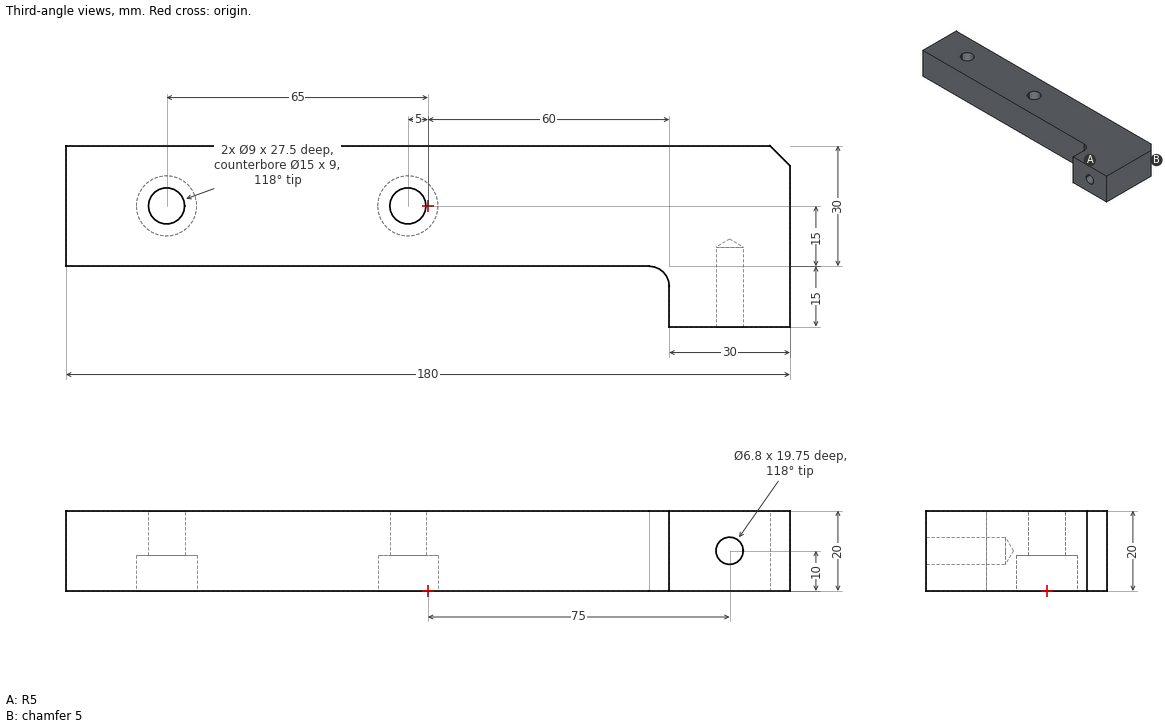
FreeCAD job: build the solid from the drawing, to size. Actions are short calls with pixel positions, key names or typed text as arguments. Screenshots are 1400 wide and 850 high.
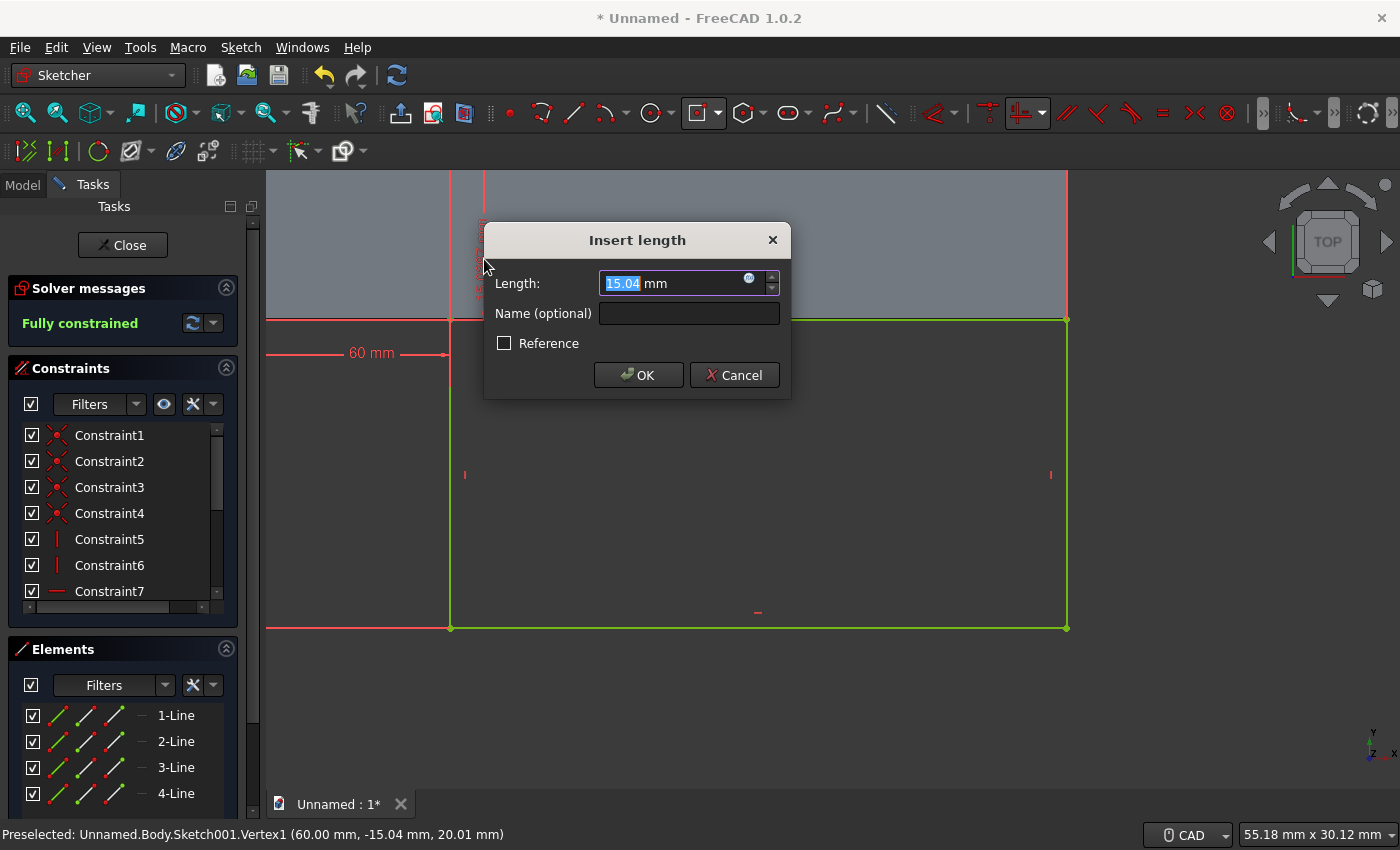
text(15)
key(Return)
key(Escape)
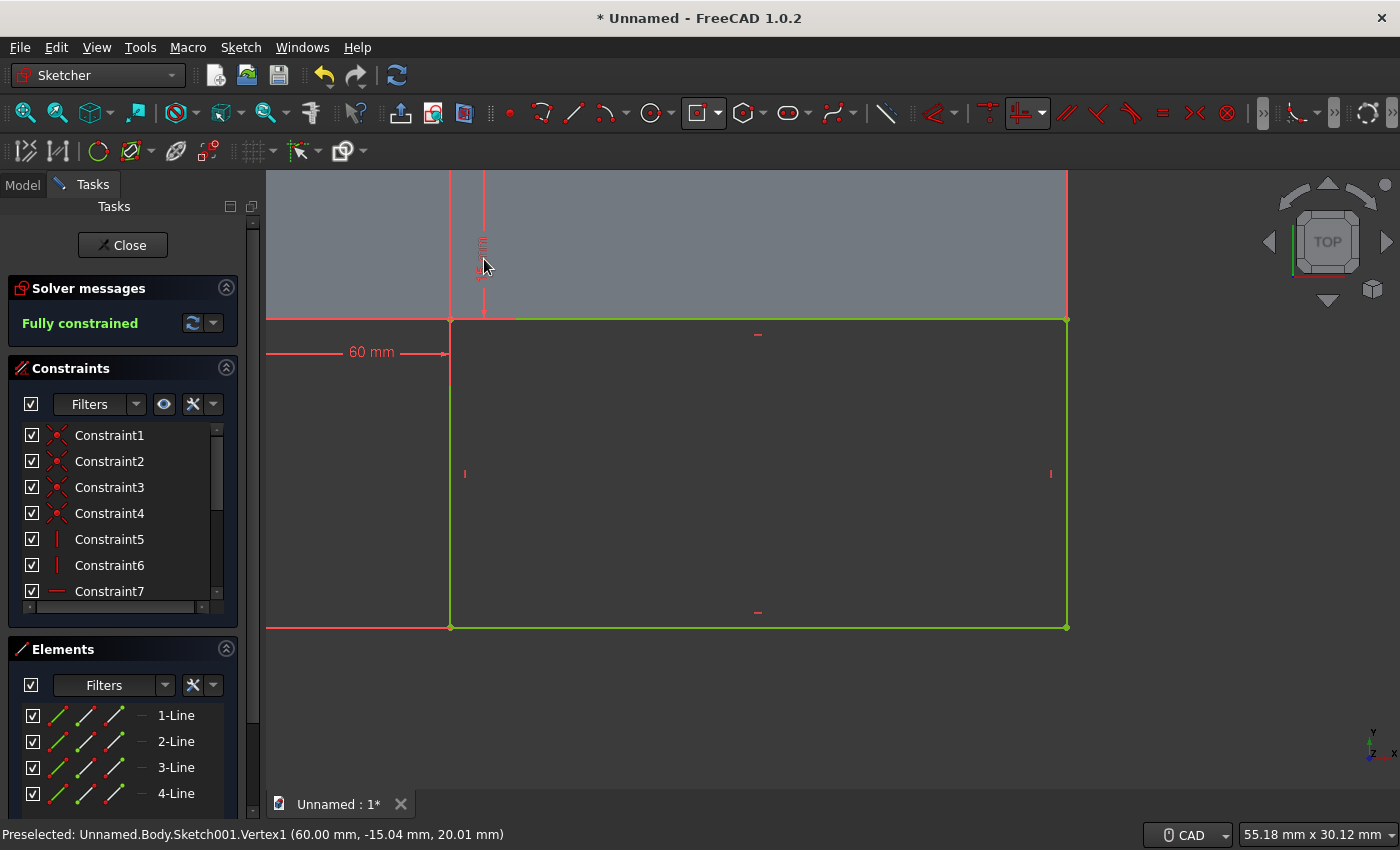
click(123, 245)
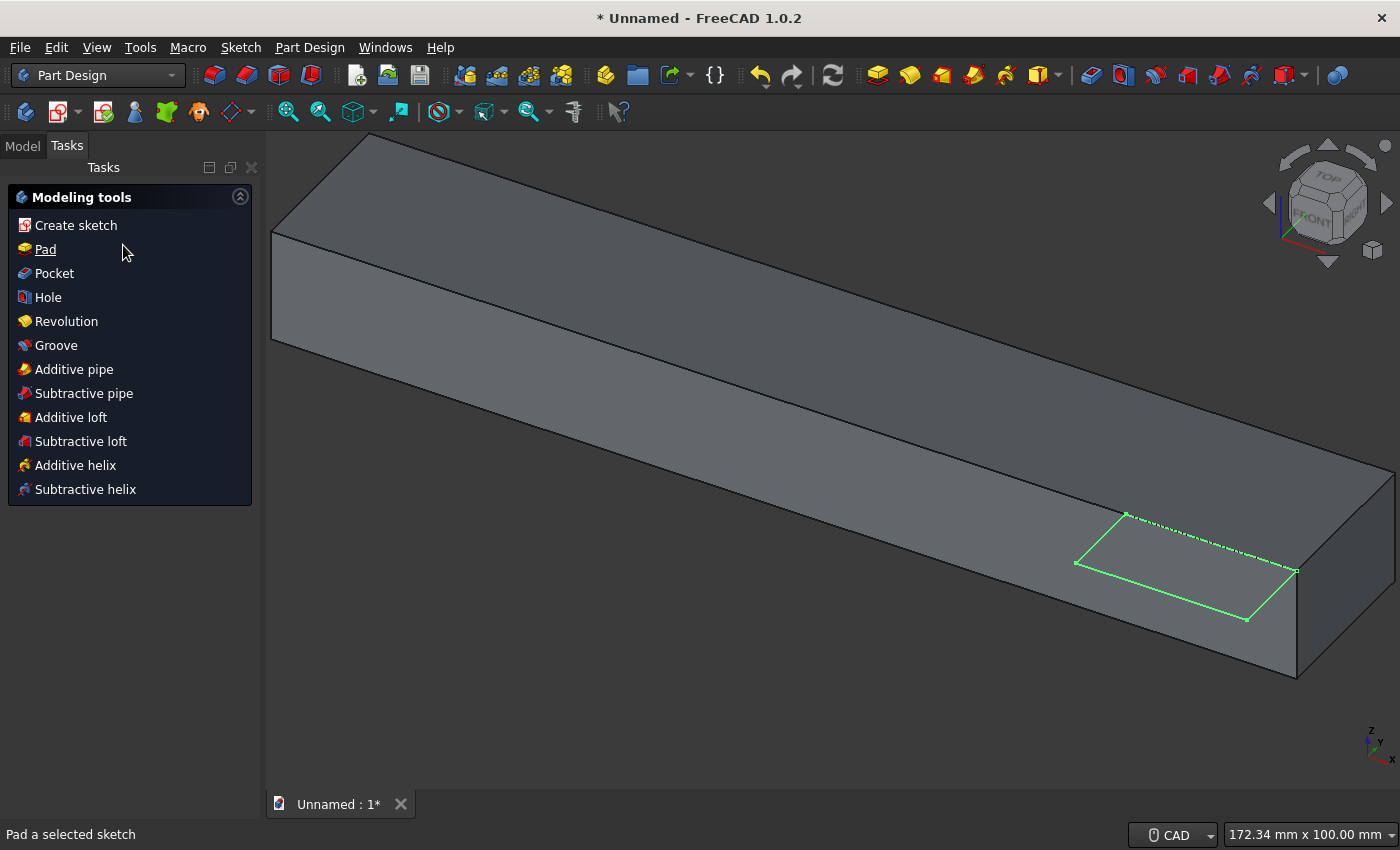
click(878, 76)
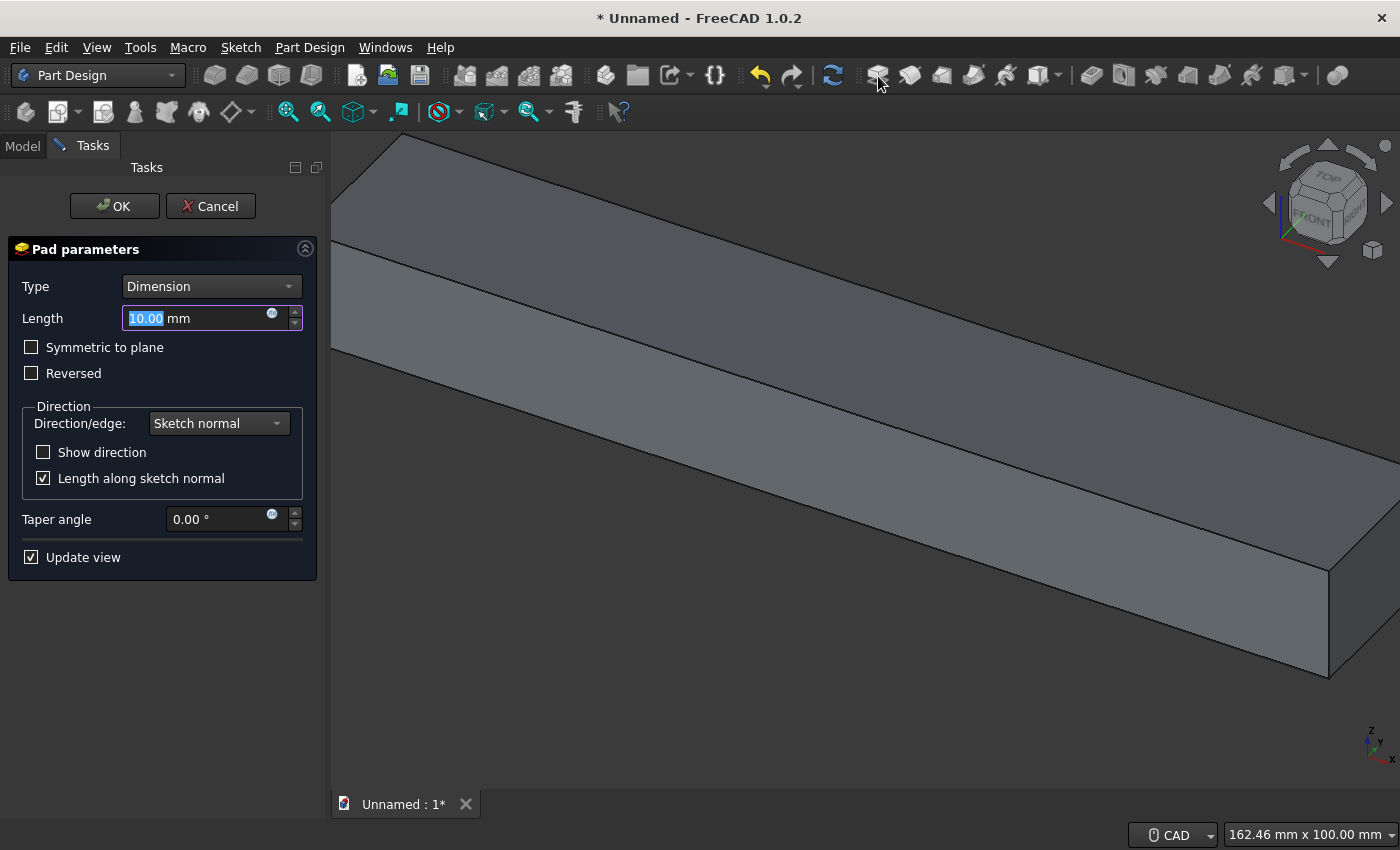
text(20)
key(Tab)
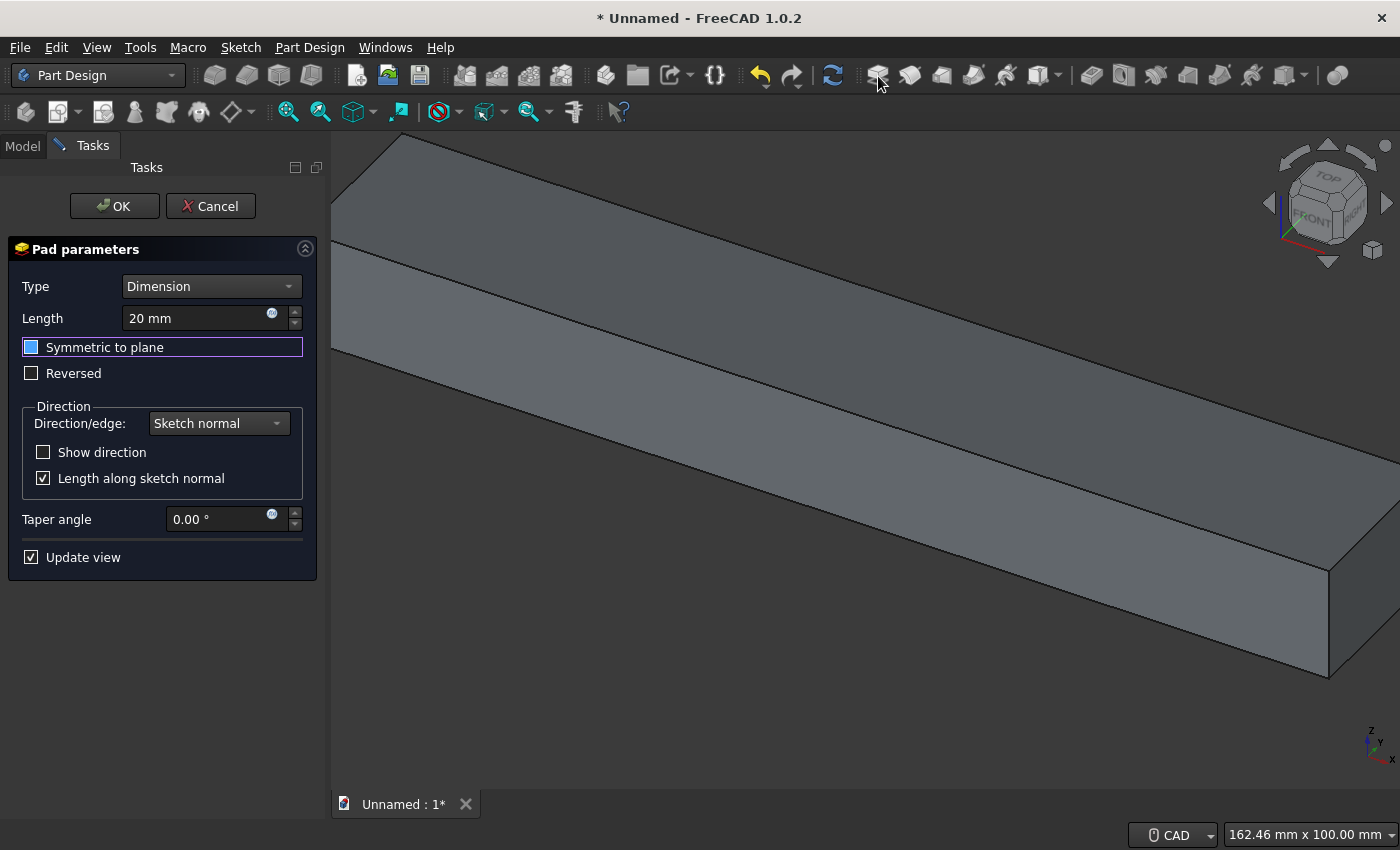
click(30, 373)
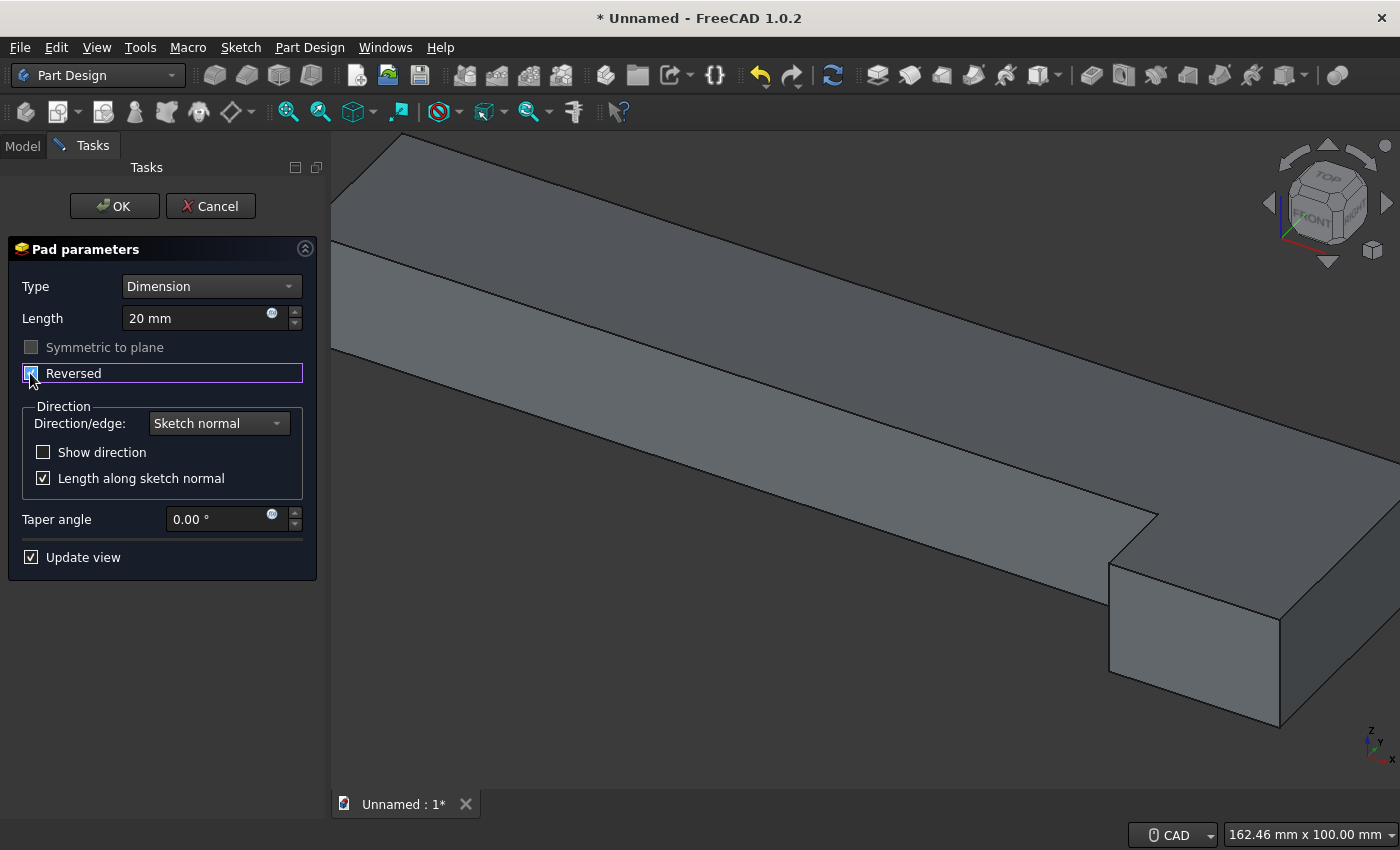
click(115, 206)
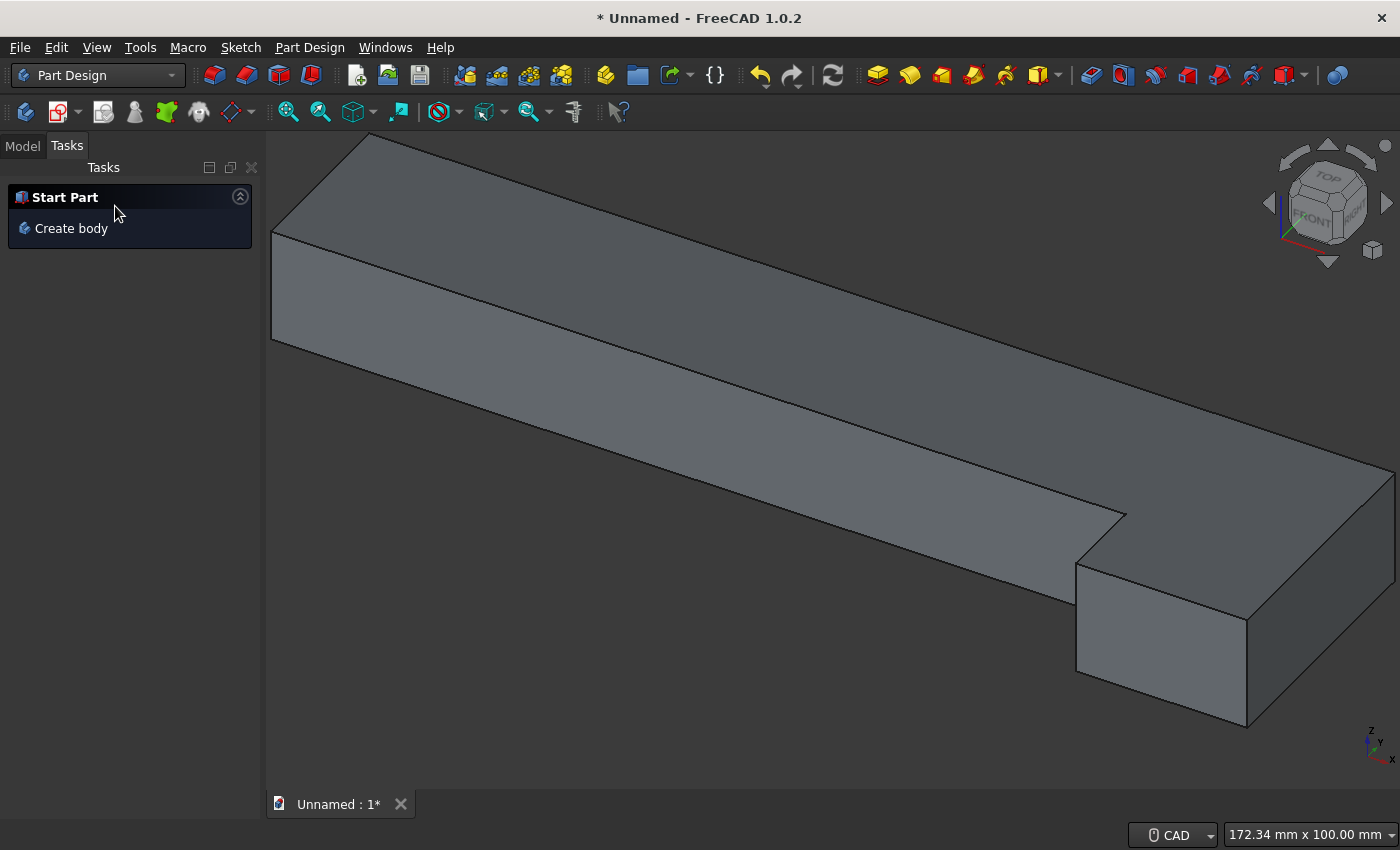
click(290, 112)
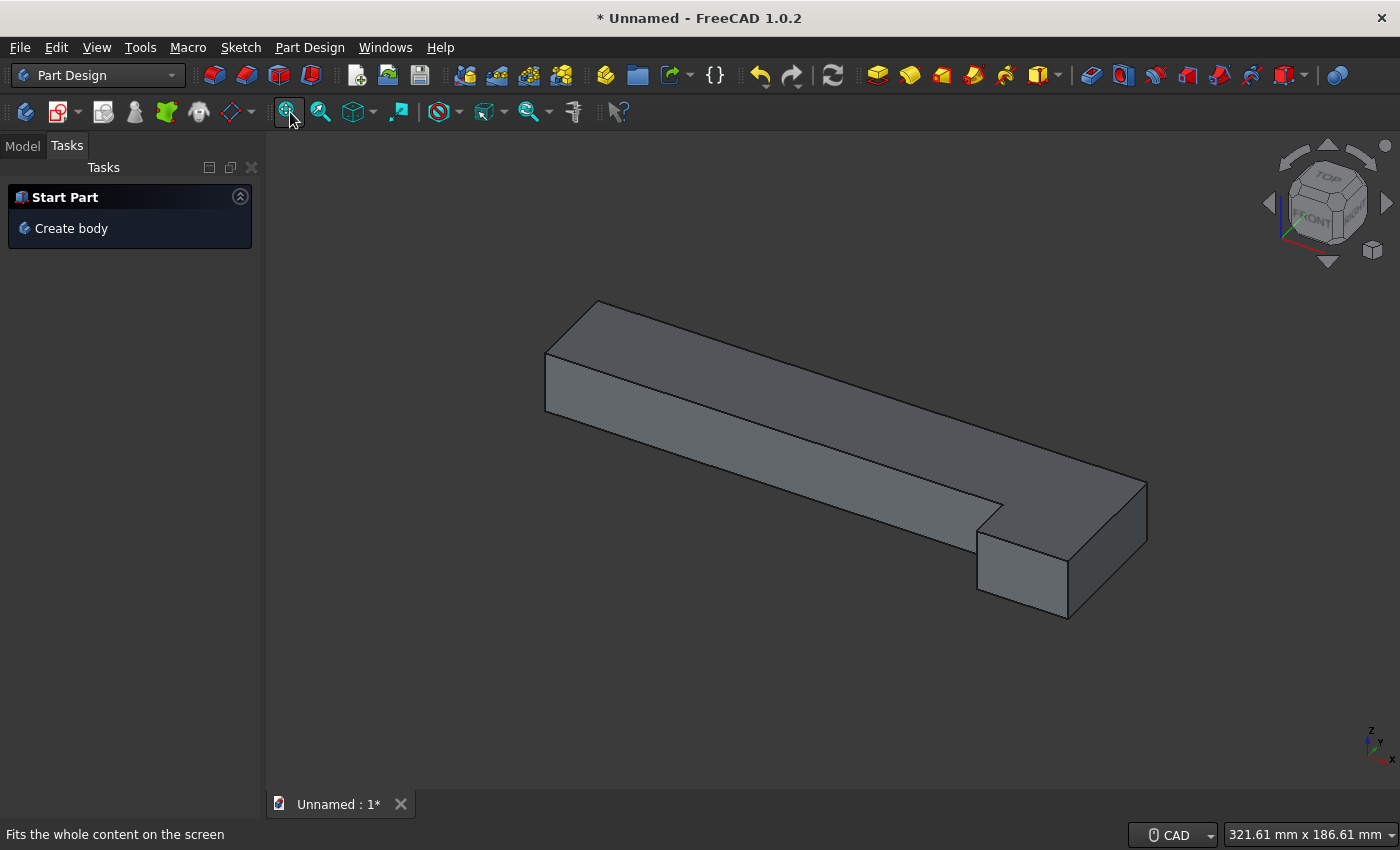
key(0)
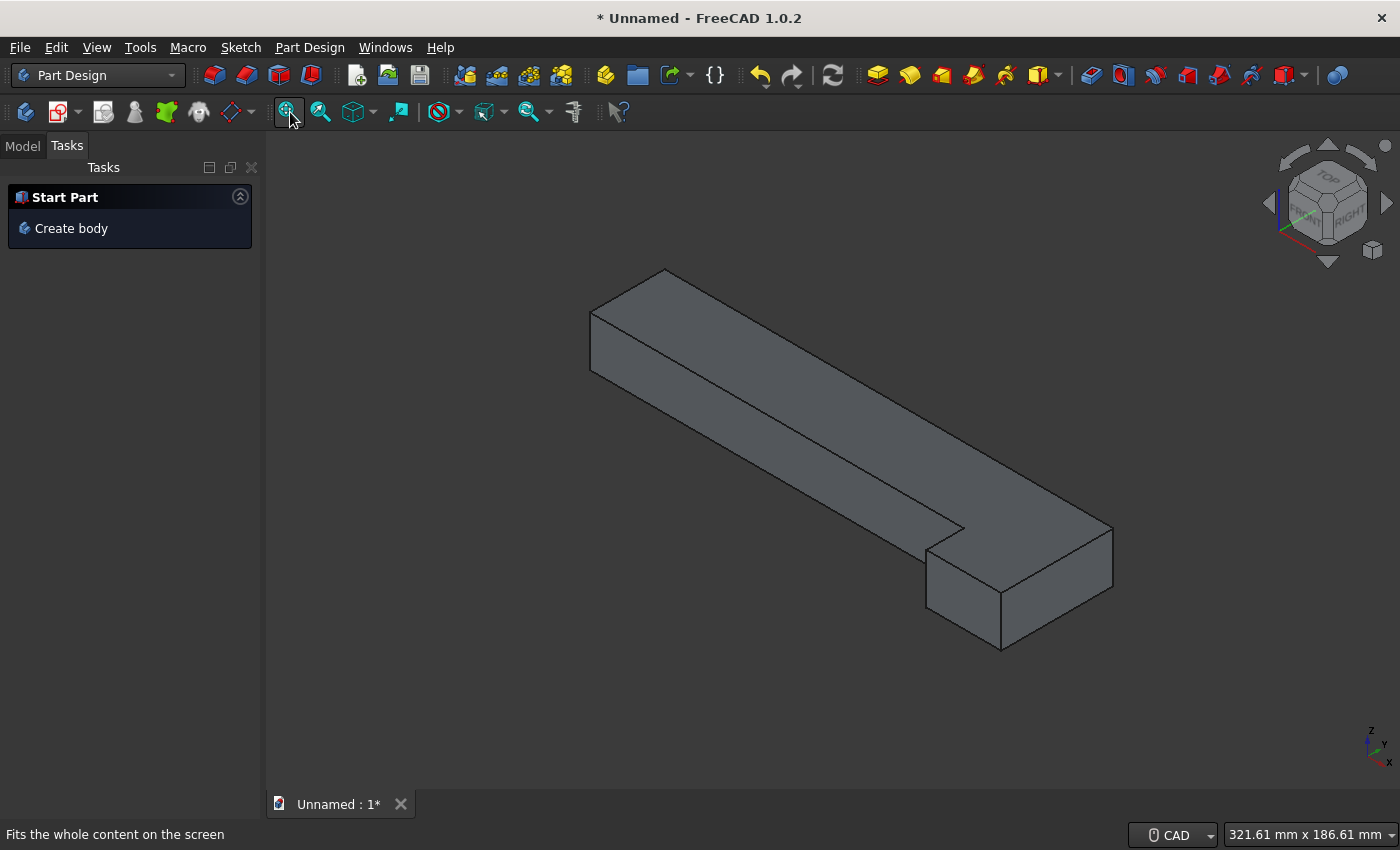
key(2)